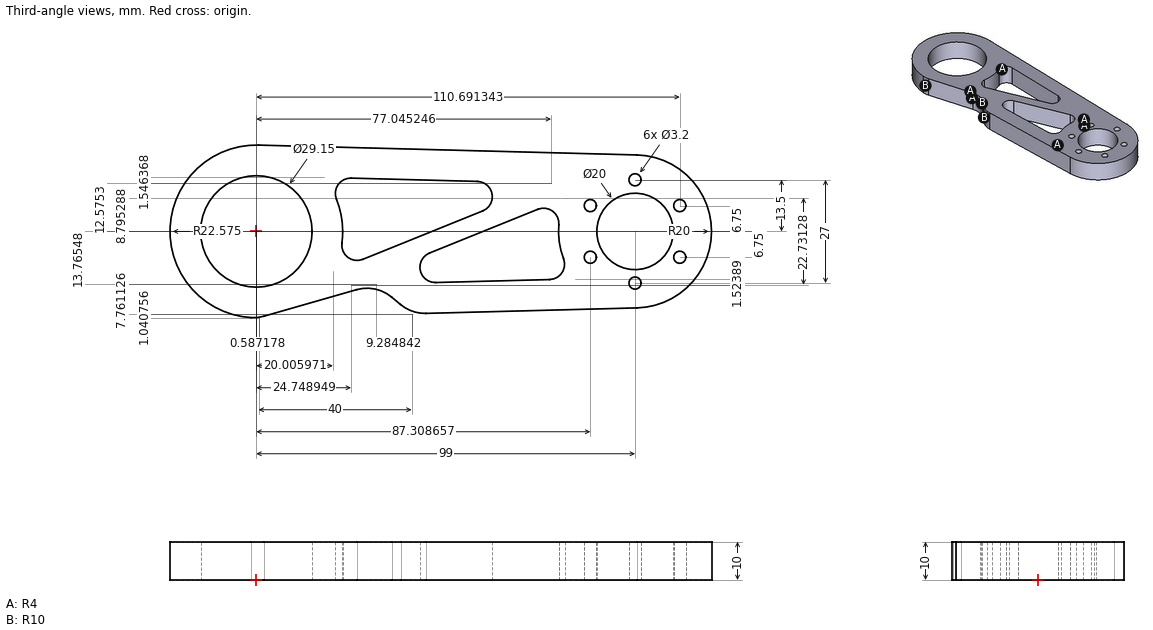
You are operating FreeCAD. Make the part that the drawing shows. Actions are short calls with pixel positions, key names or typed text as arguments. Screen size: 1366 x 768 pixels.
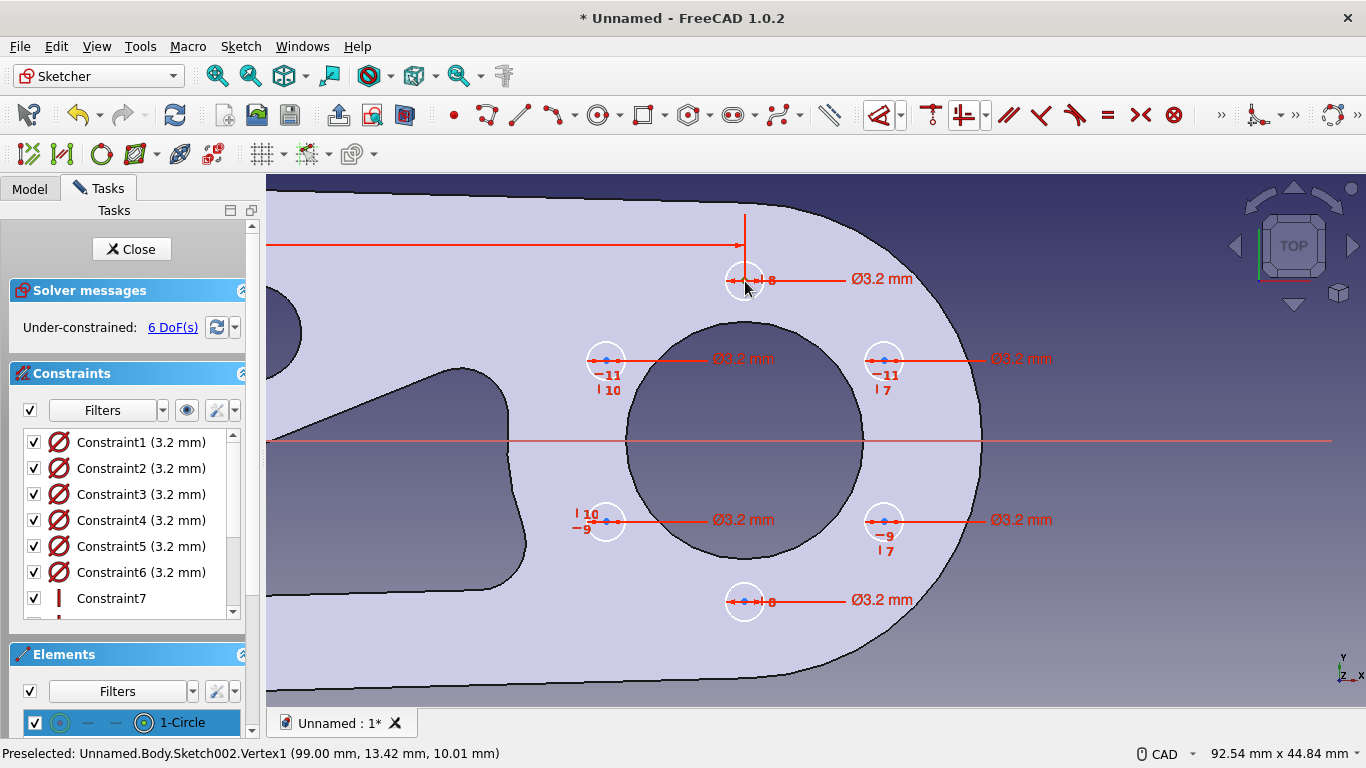
click(745, 602)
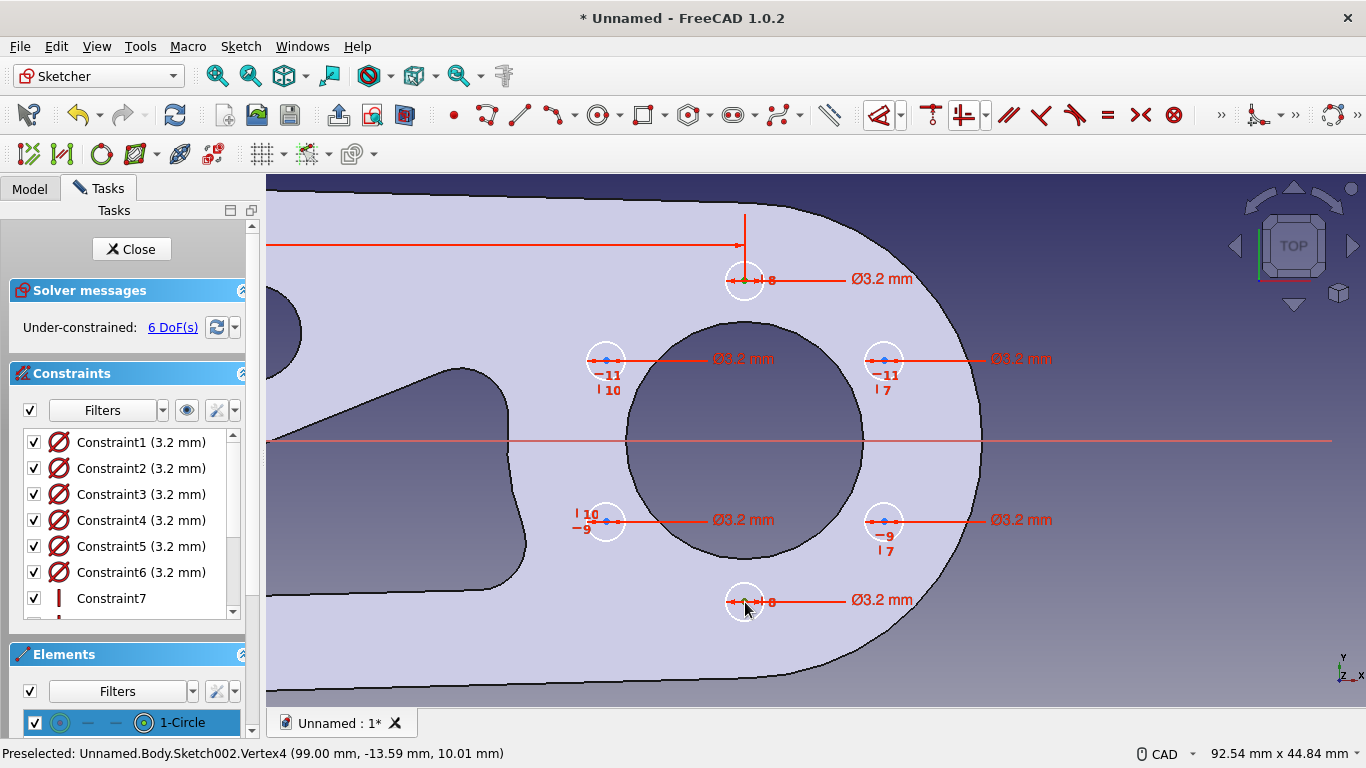
key(i)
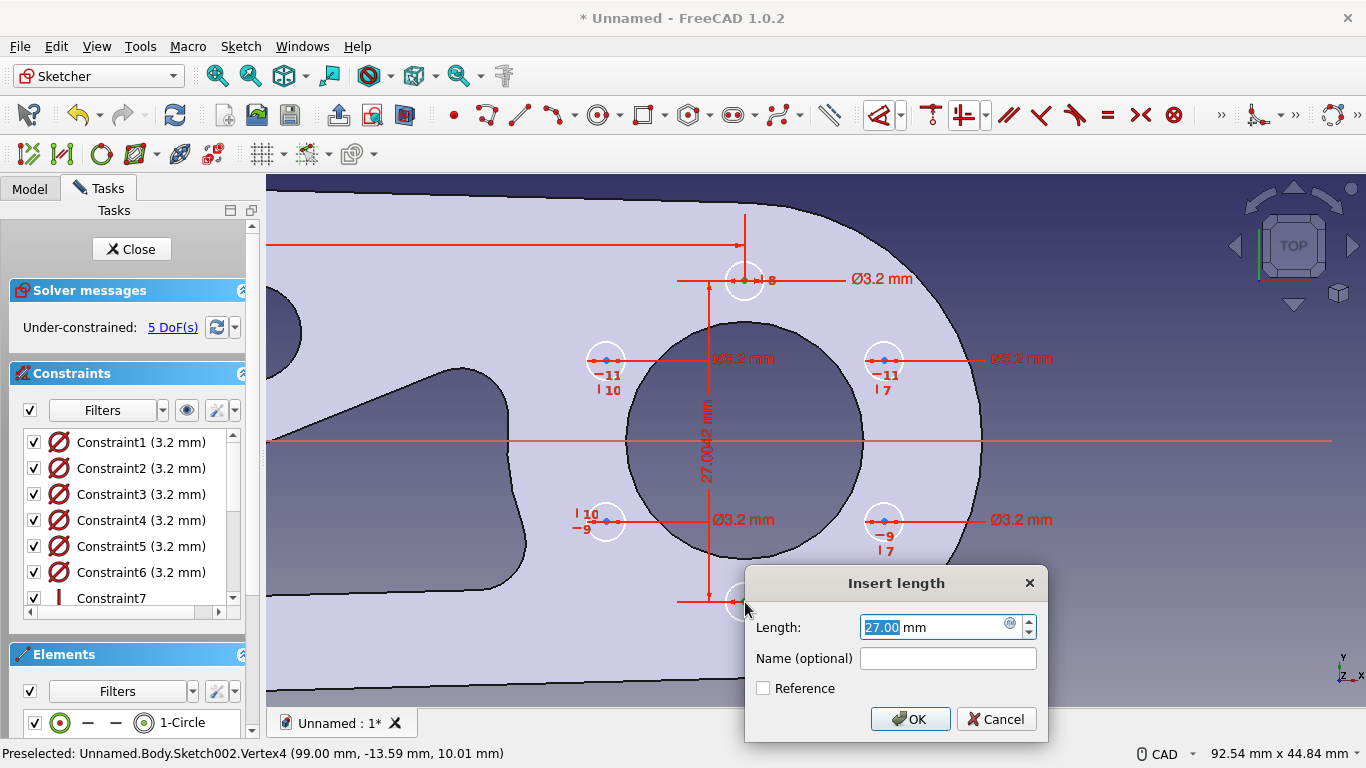
text(27)
key(Return)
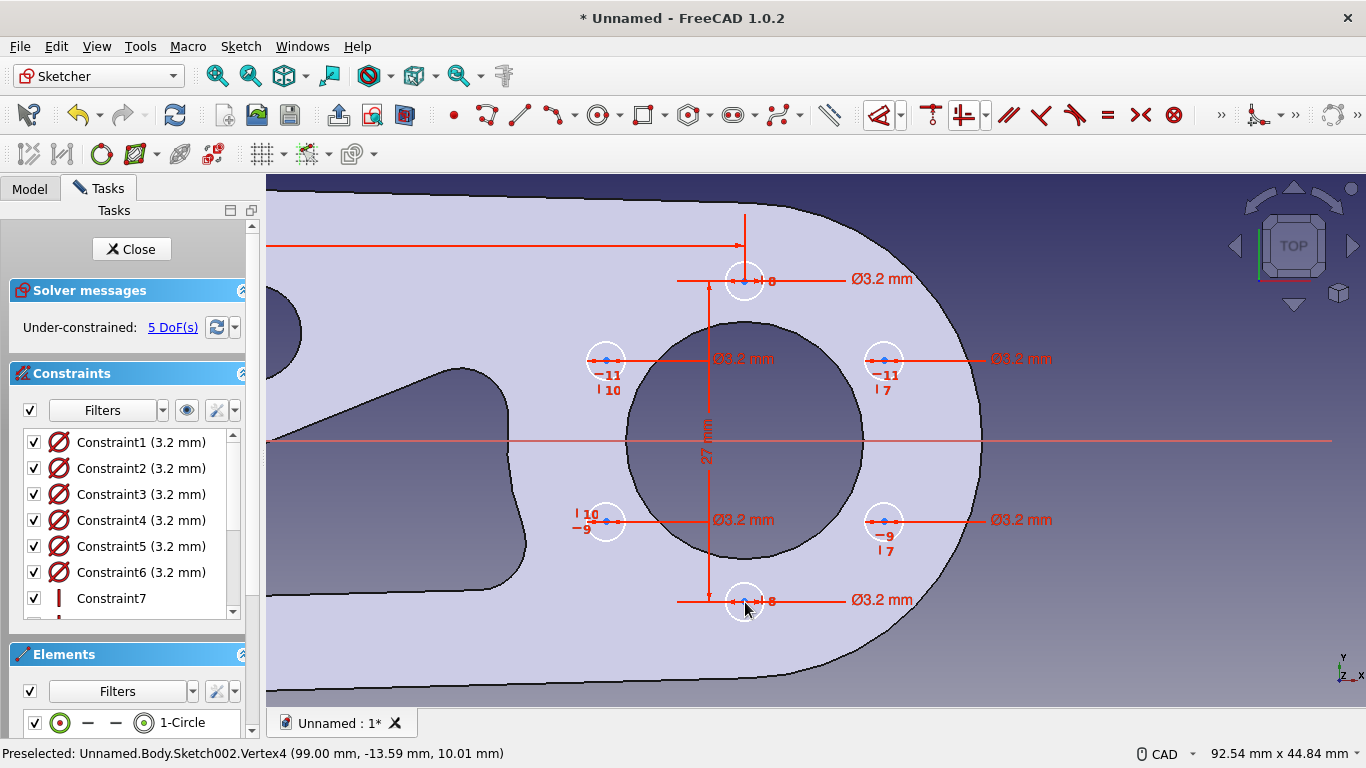
click(745, 281)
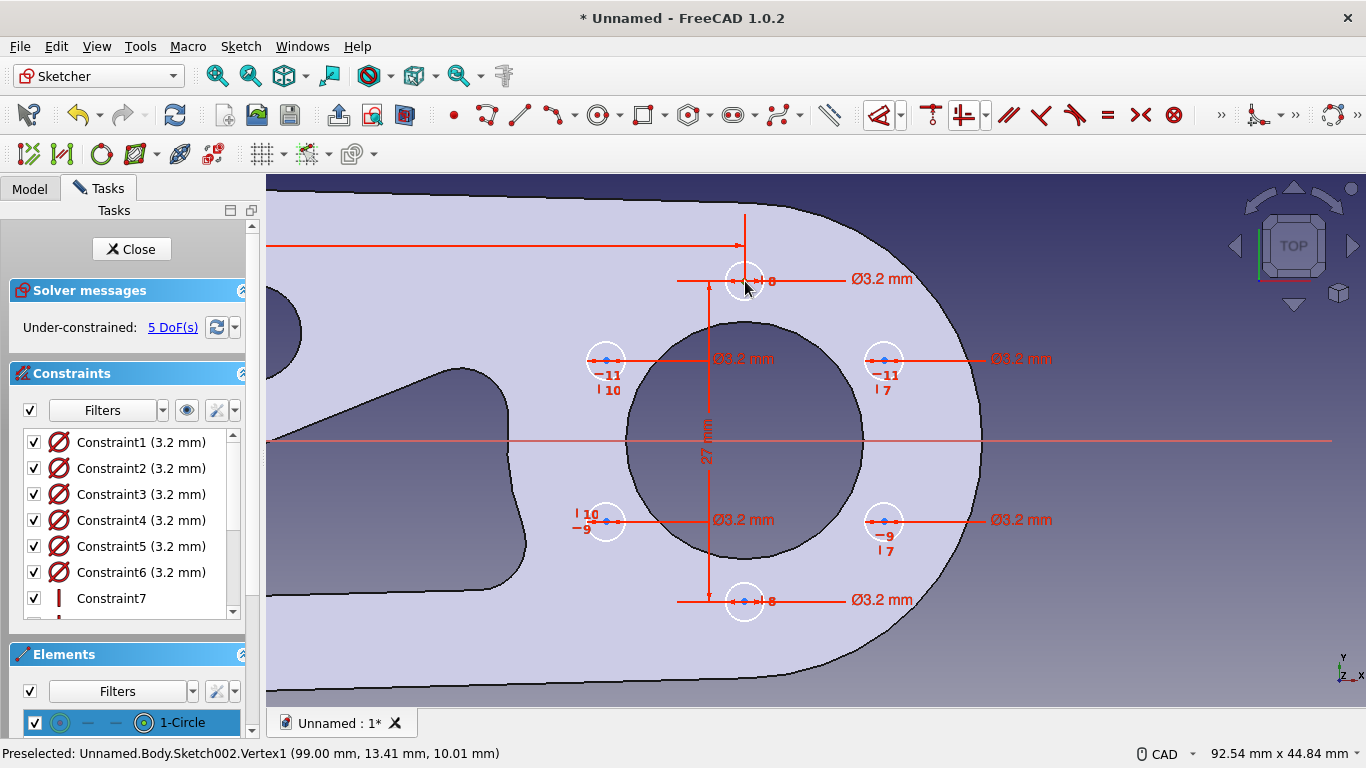
click(900, 116)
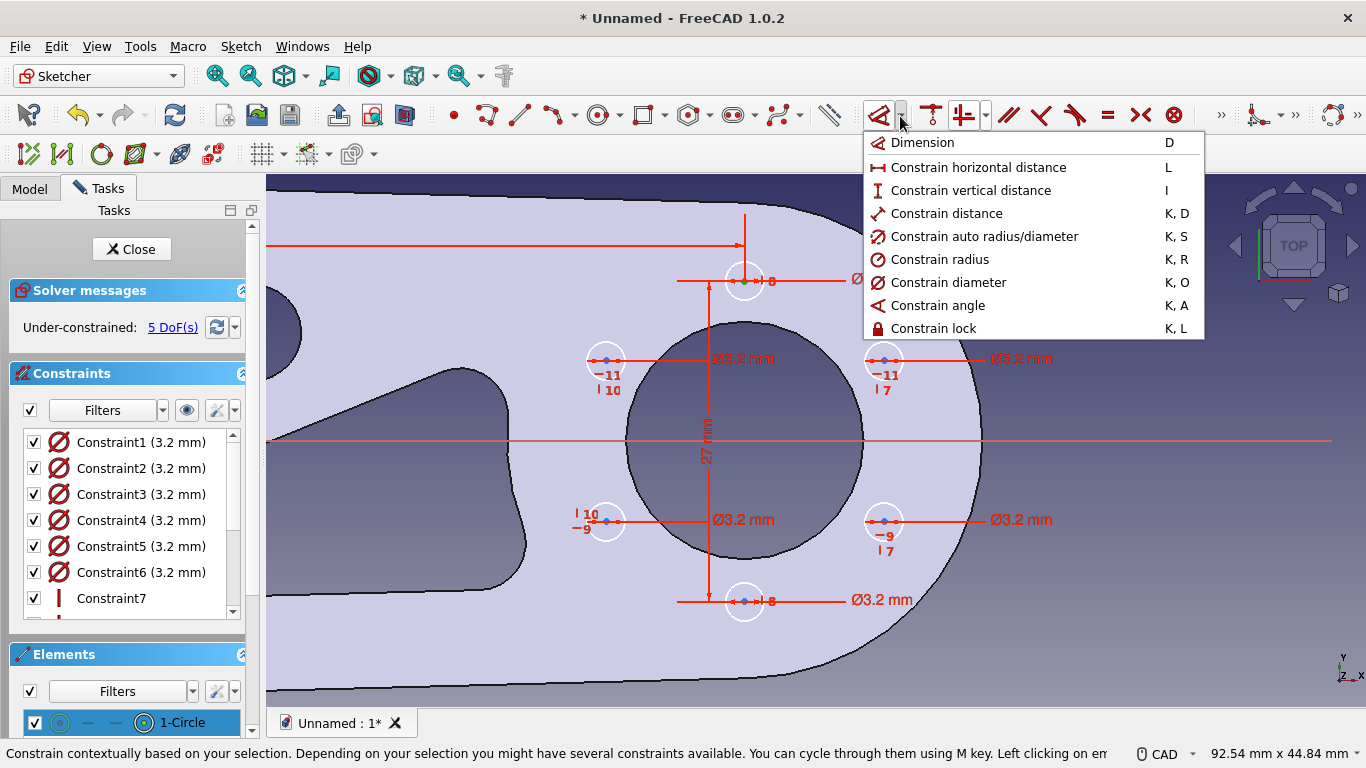
click(1034, 190)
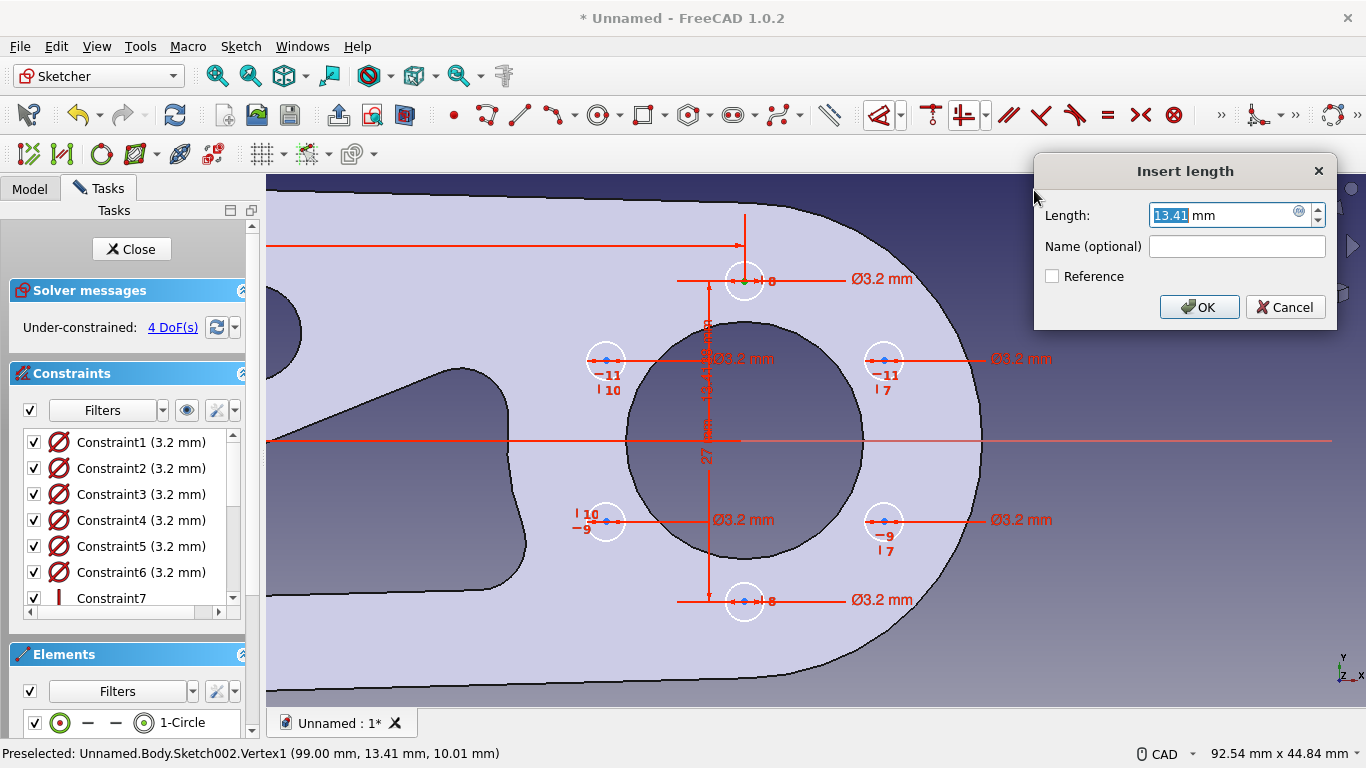
text(13.5)
key(Return)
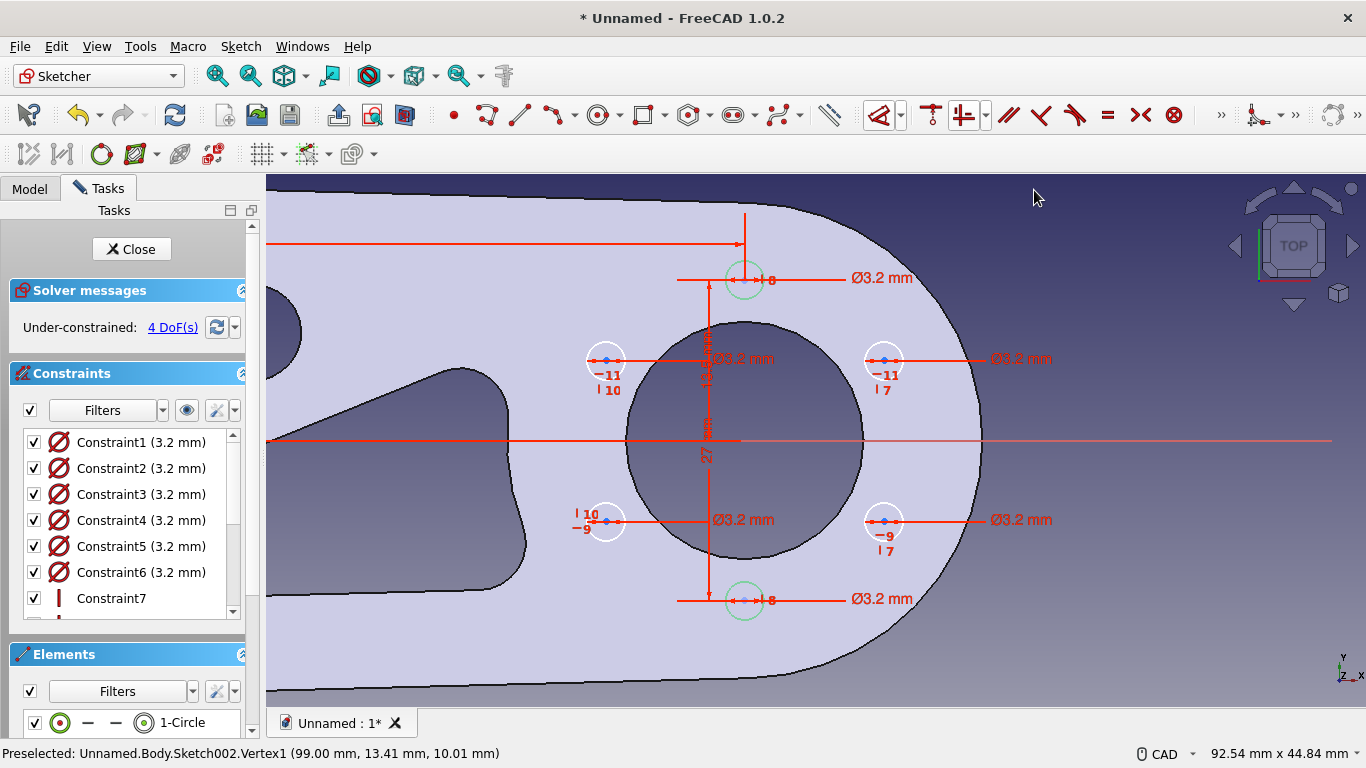
click(884, 361)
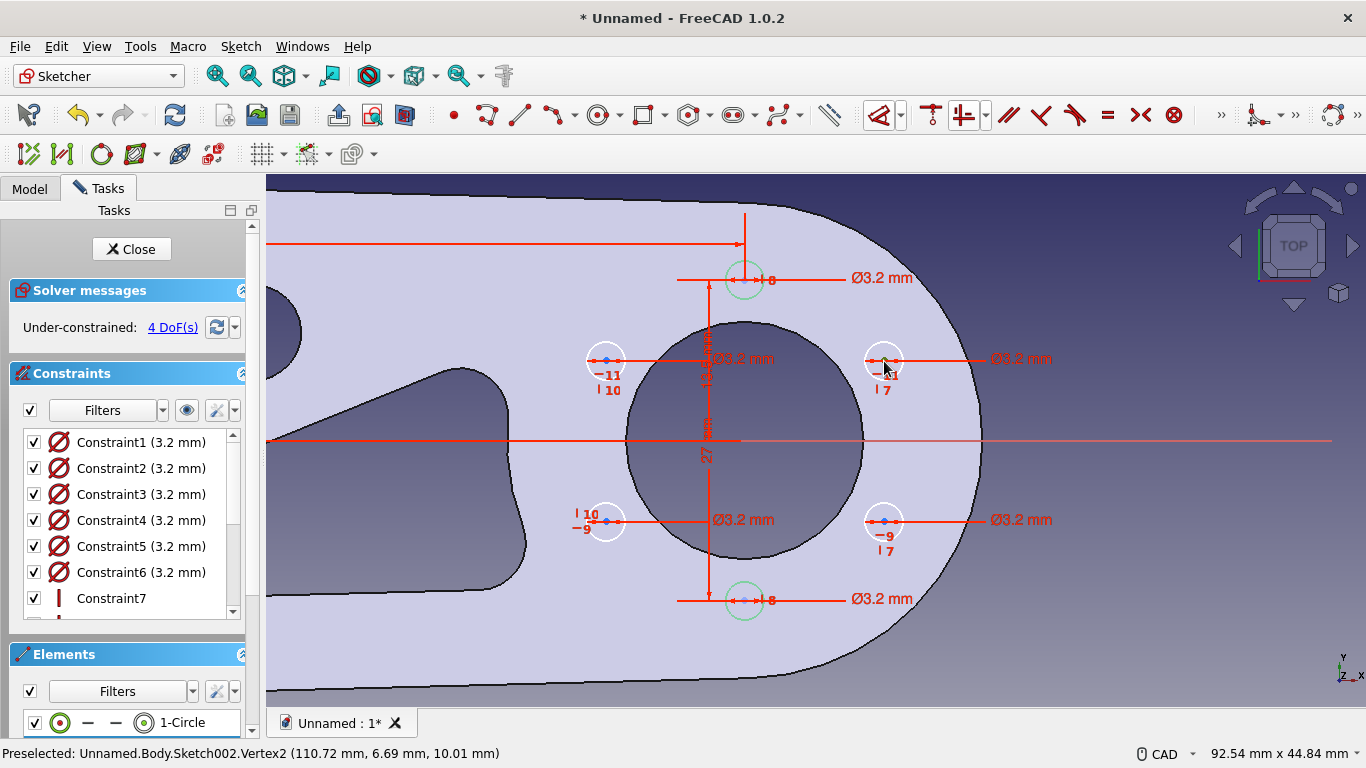
key(i)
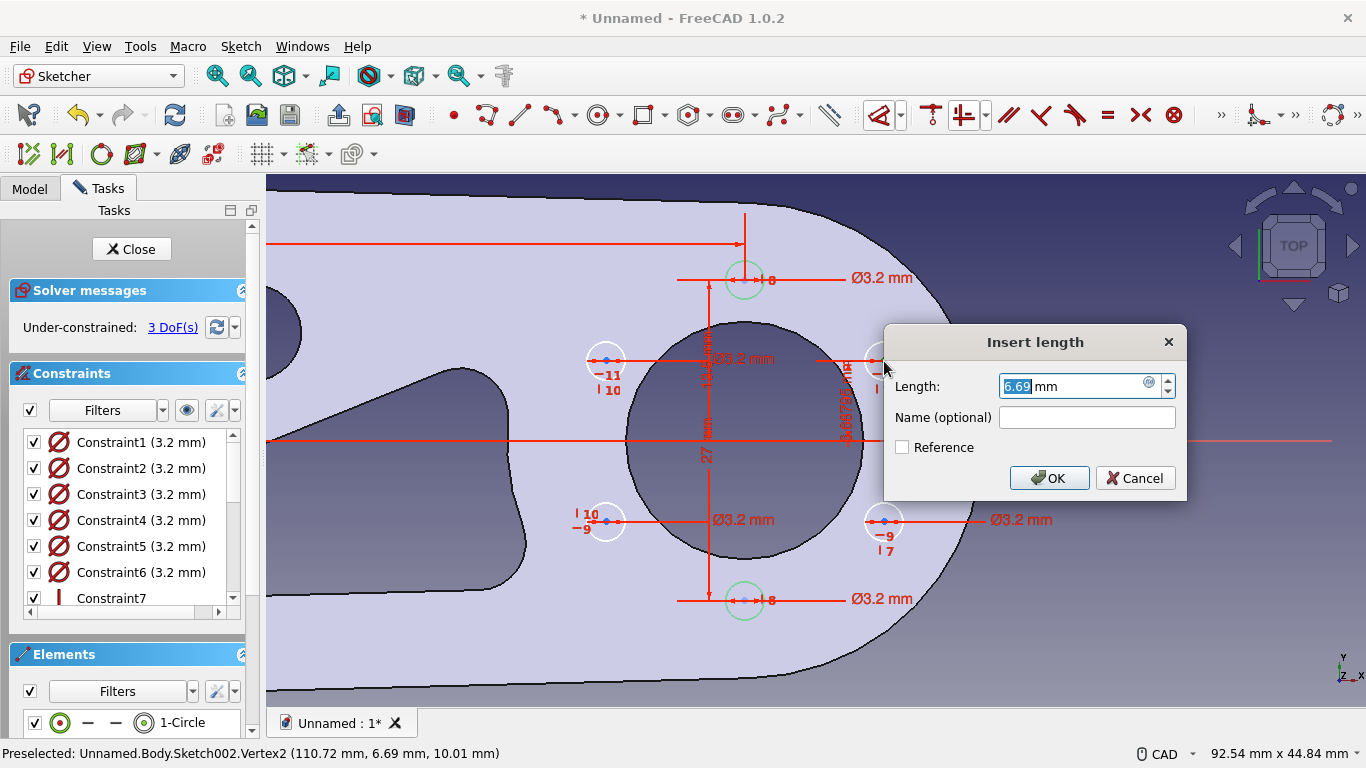
text(6.75)
key(Return)